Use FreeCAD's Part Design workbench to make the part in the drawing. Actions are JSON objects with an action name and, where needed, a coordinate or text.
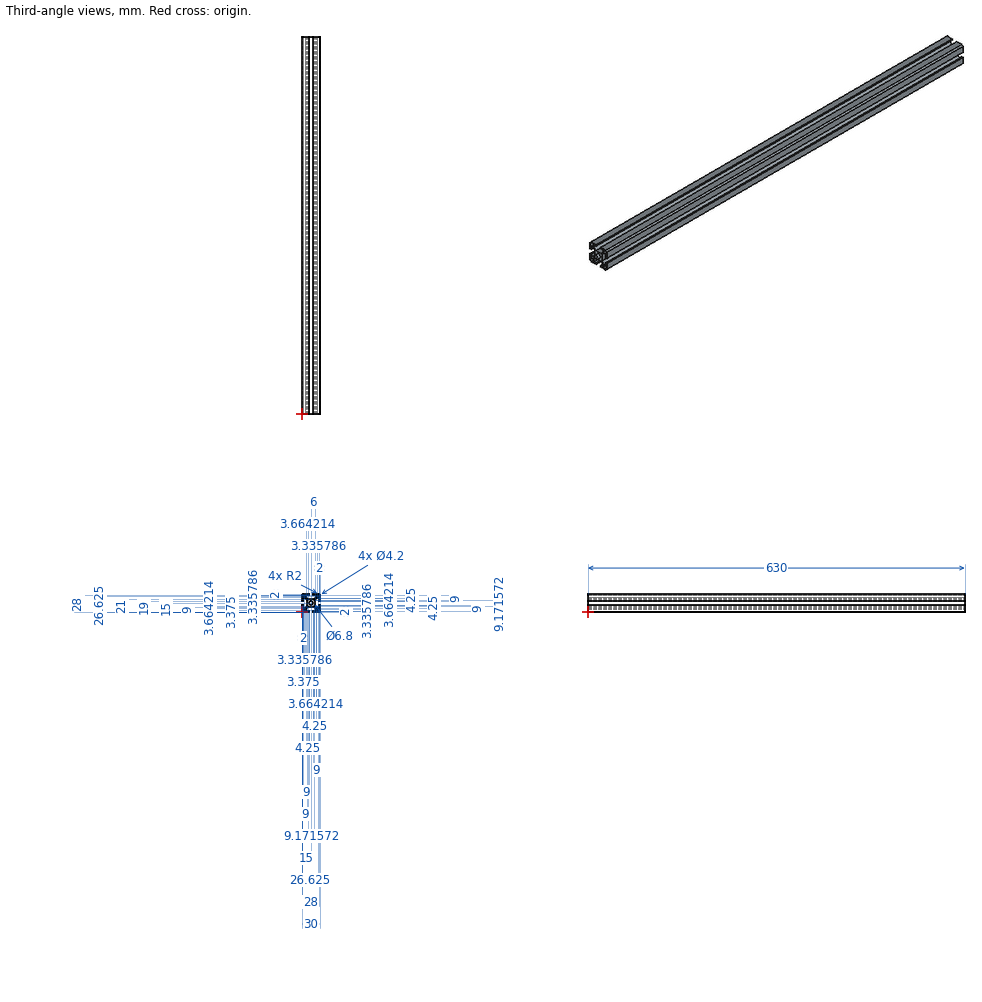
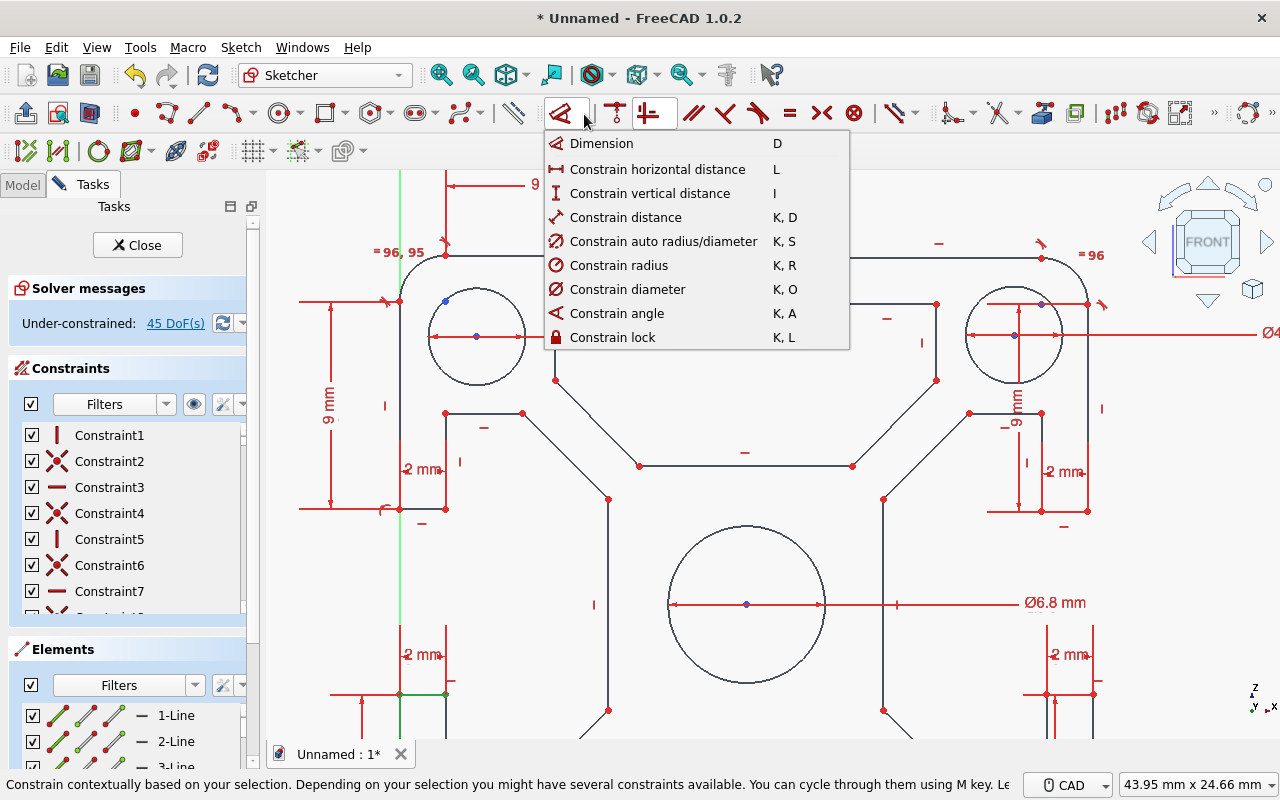
{"action": "left_click", "coordinate": [697, 193]}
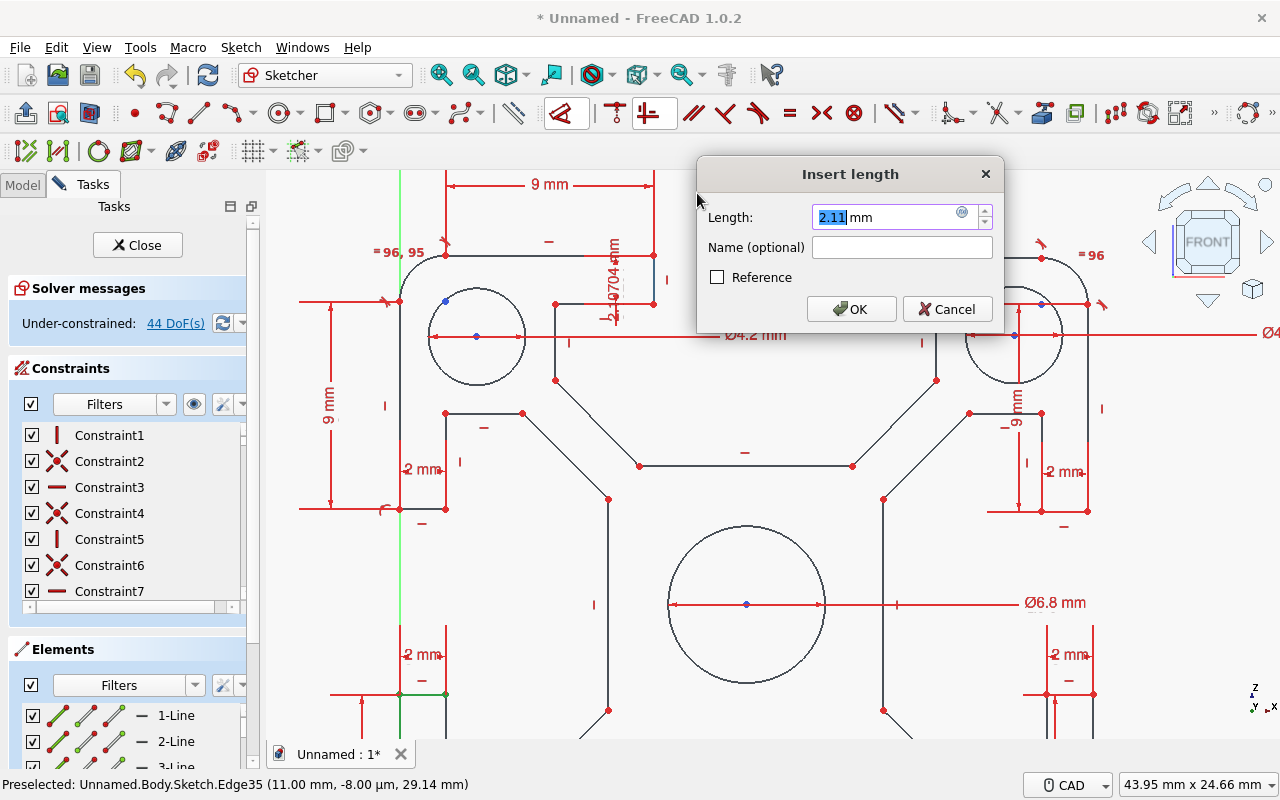
{"action": "type", "text": "2"}
{"action": "key", "text": "Return"}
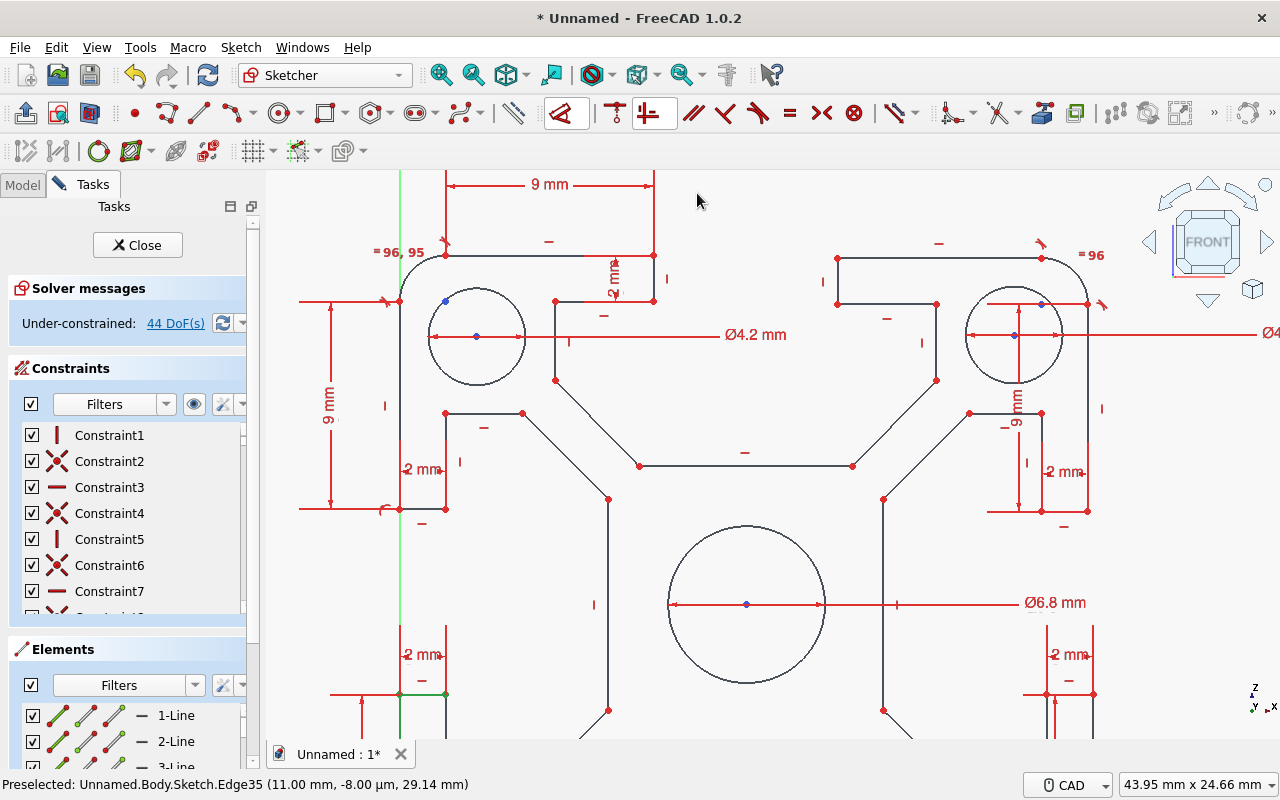
{"action": "left_click", "coordinate": [838, 290]}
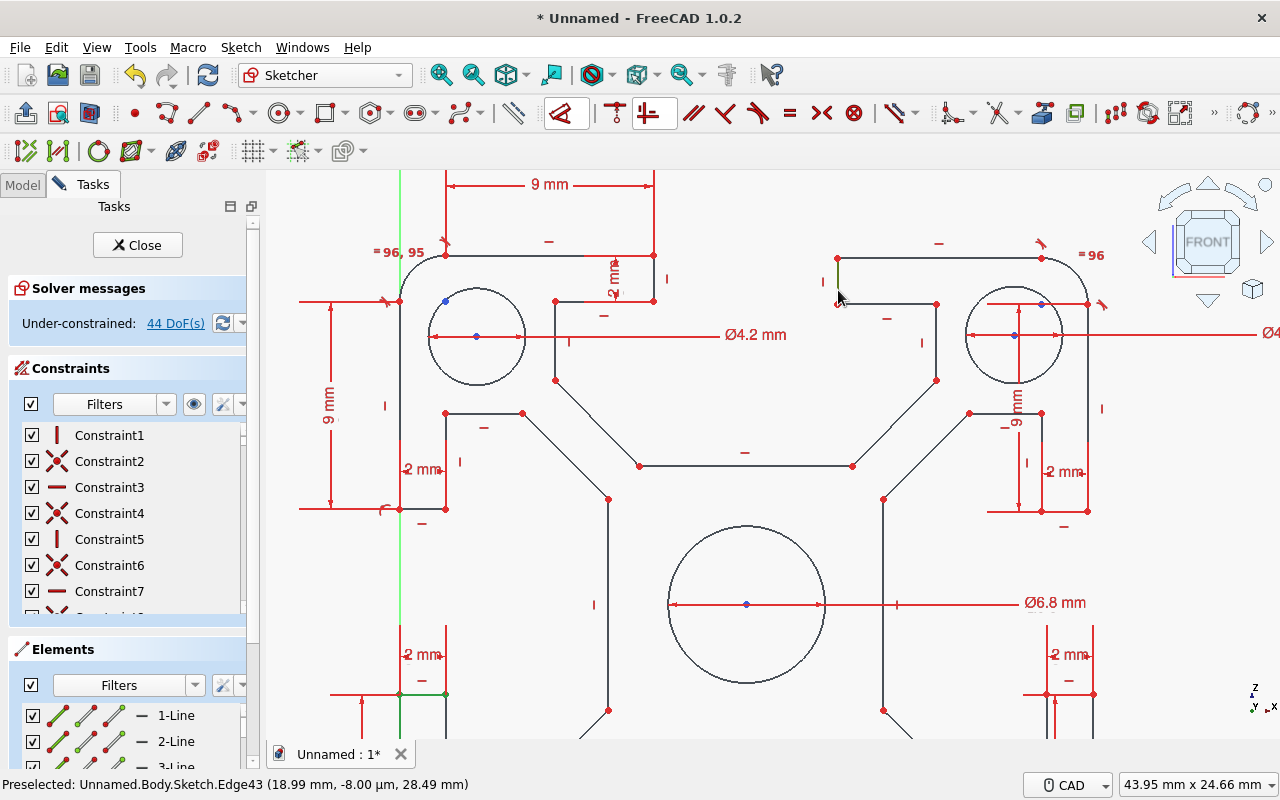
{"action": "key", "text": "i"}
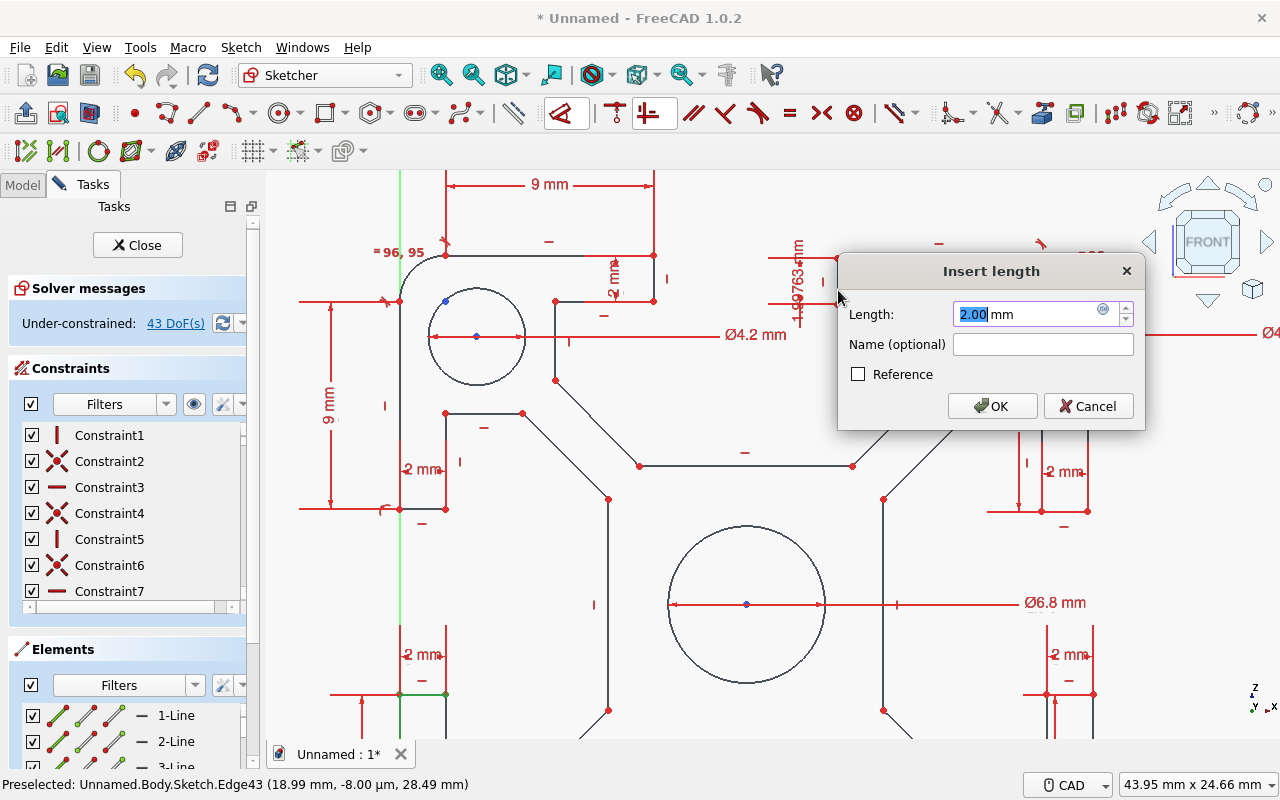
{"action": "type", "text": "2"}
{"action": "key", "text": "Return"}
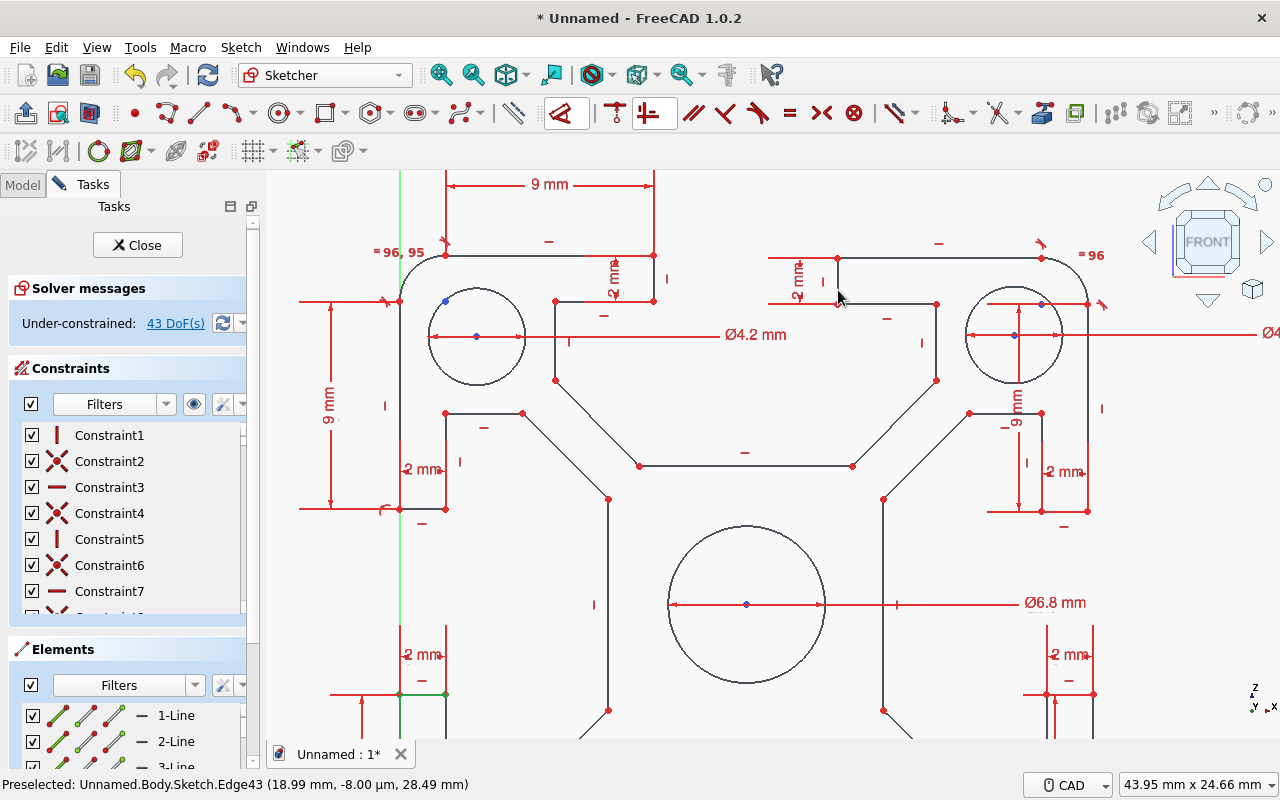
{"action": "left_click", "coordinate": [899, 258]}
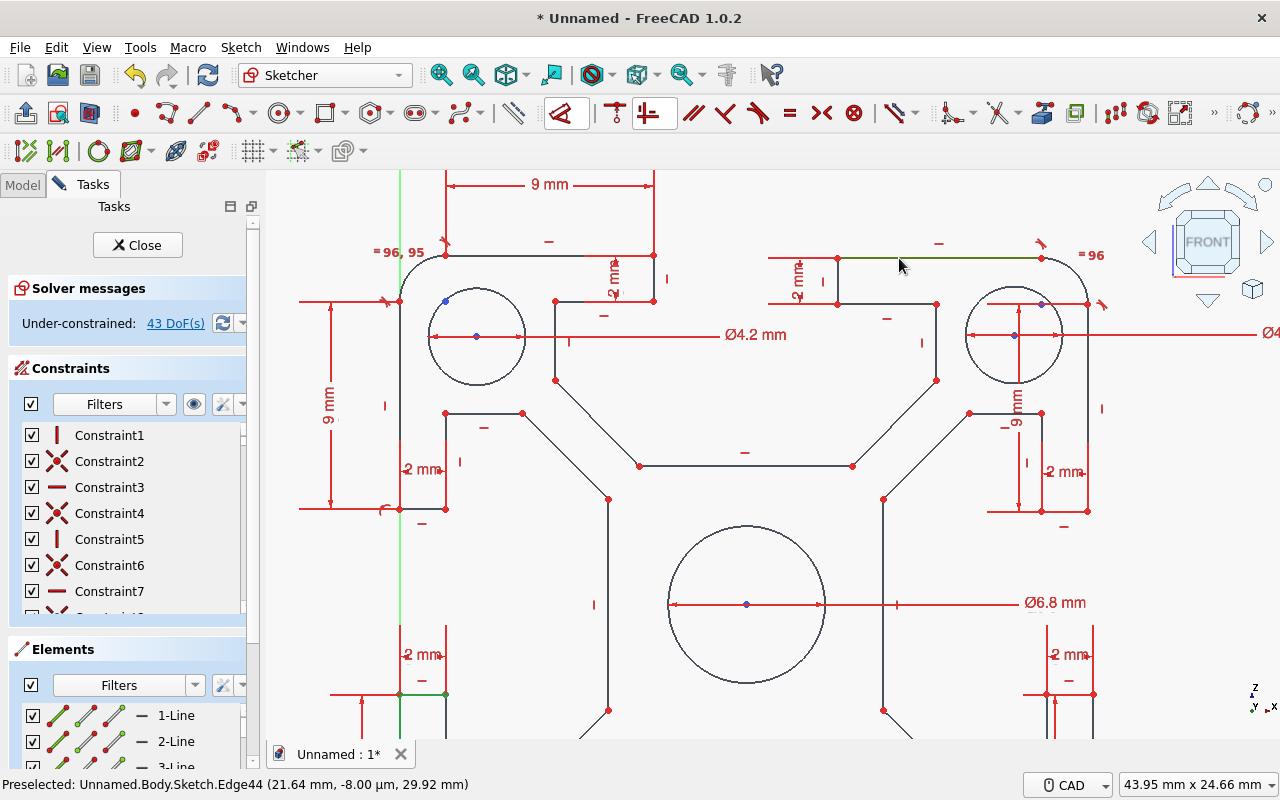
{"action": "left_click", "coordinate": [584, 114]}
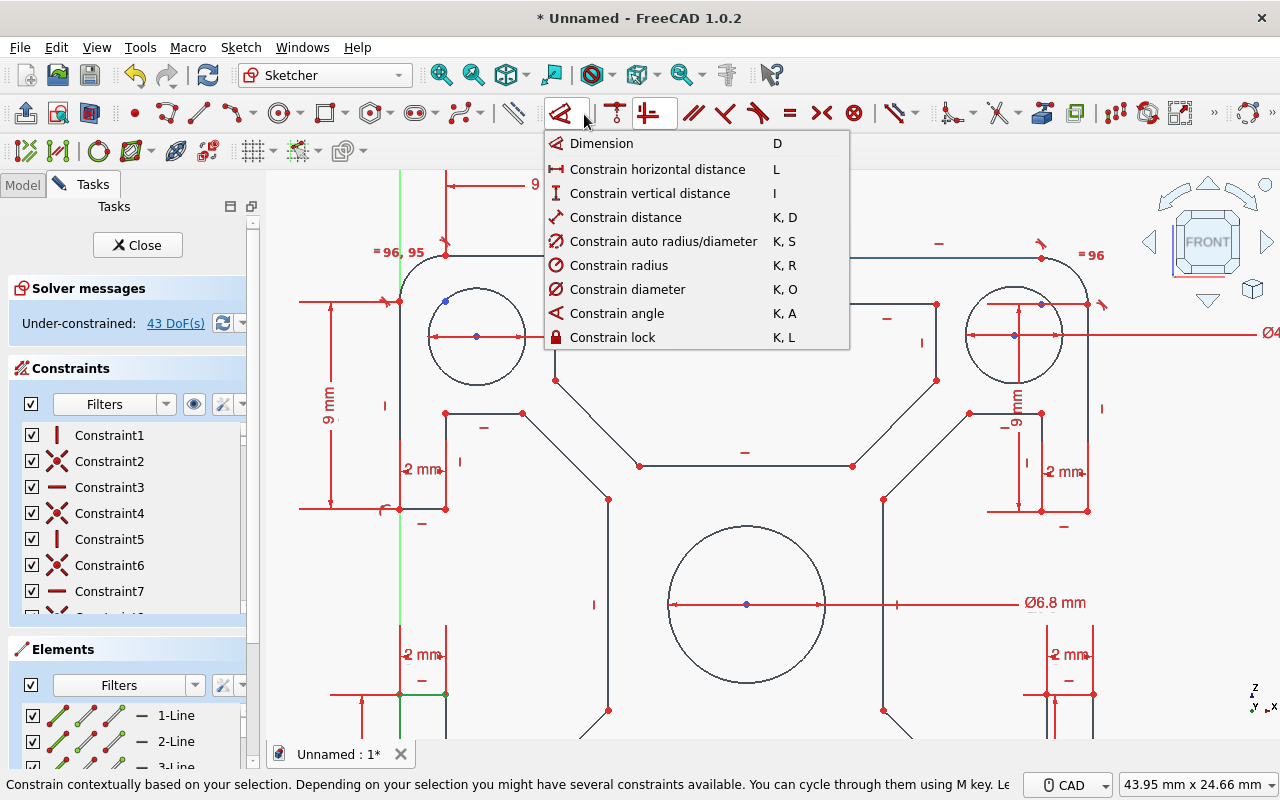
{"action": "left_click", "coordinate": [697, 169]}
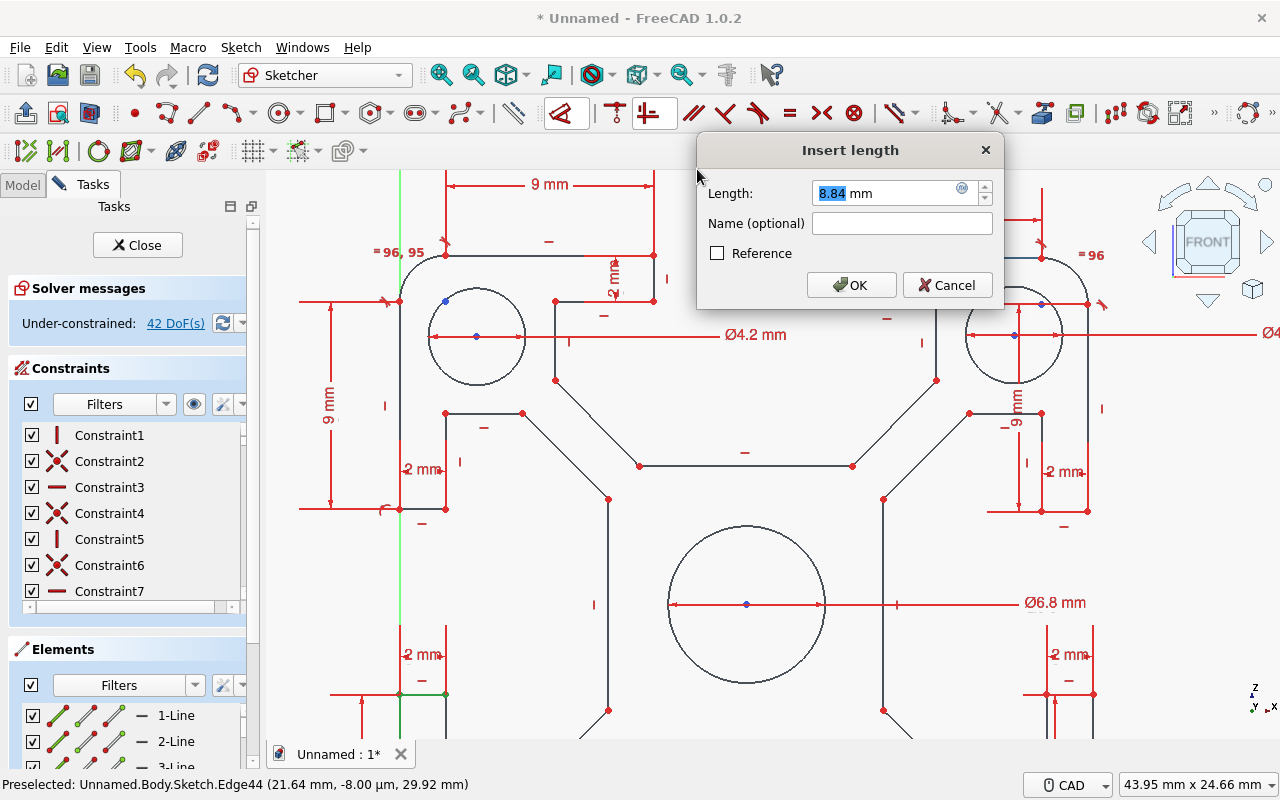
{"action": "type", "text": "9"}
{"action": "key", "text": "Return"}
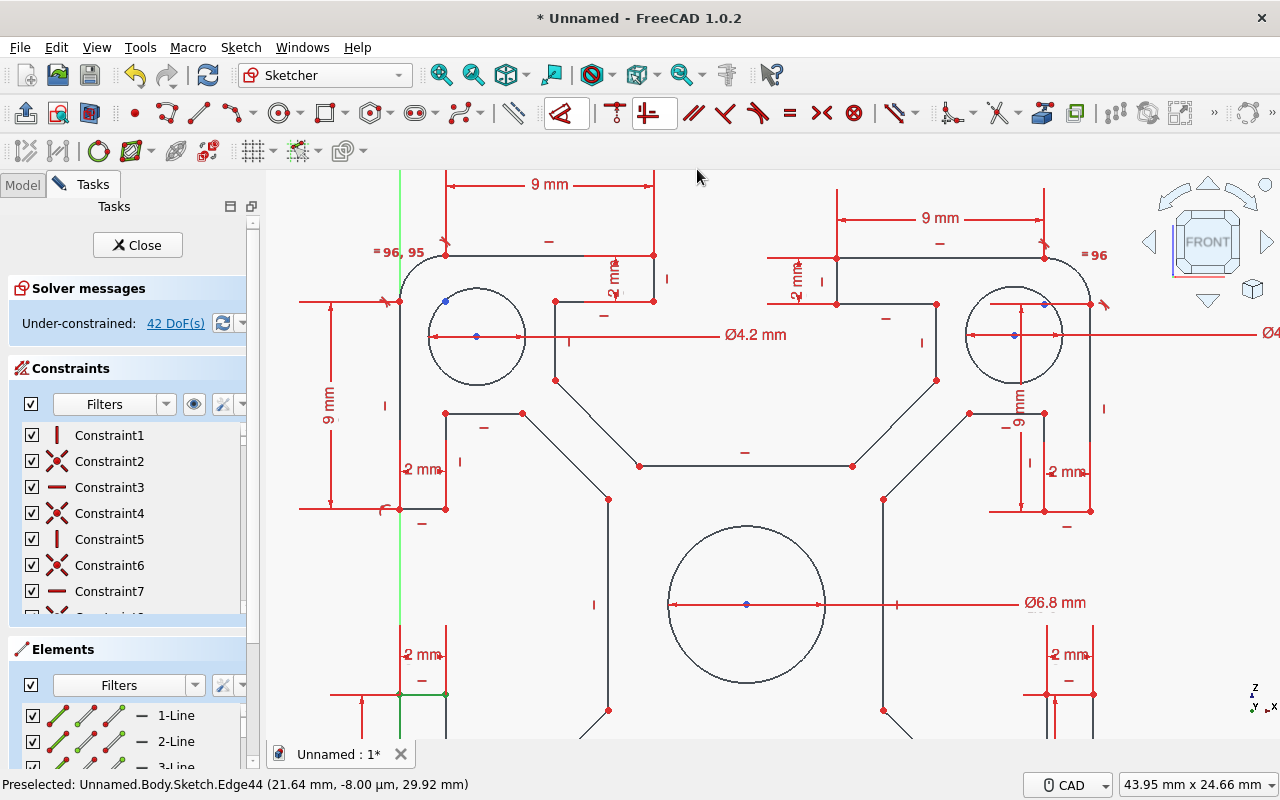
{"action": "scroll", "coordinate": [654, 275], "scroll_direction": "down", "scroll_amount": 3}